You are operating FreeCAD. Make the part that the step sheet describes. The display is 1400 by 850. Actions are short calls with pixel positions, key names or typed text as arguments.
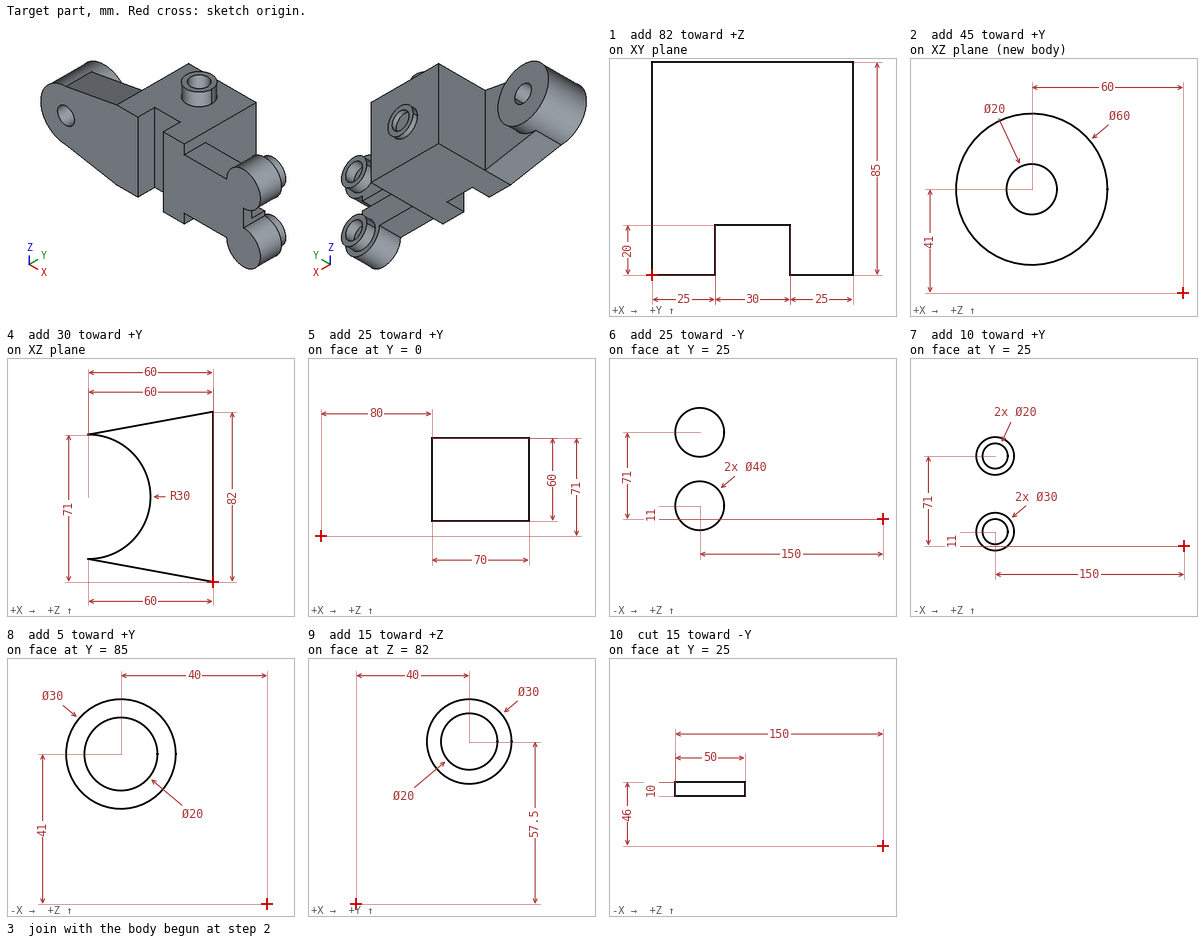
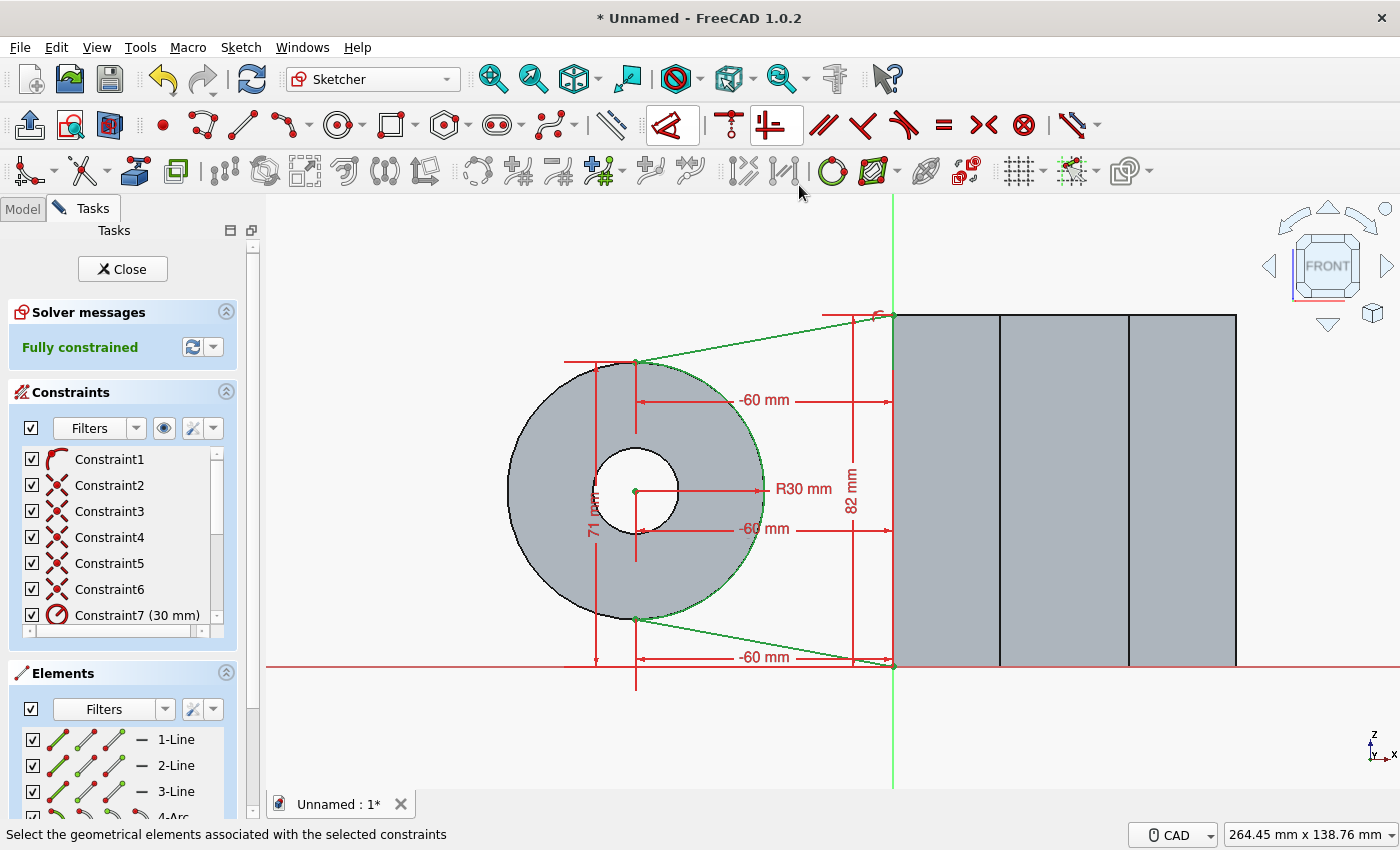
click(123, 269)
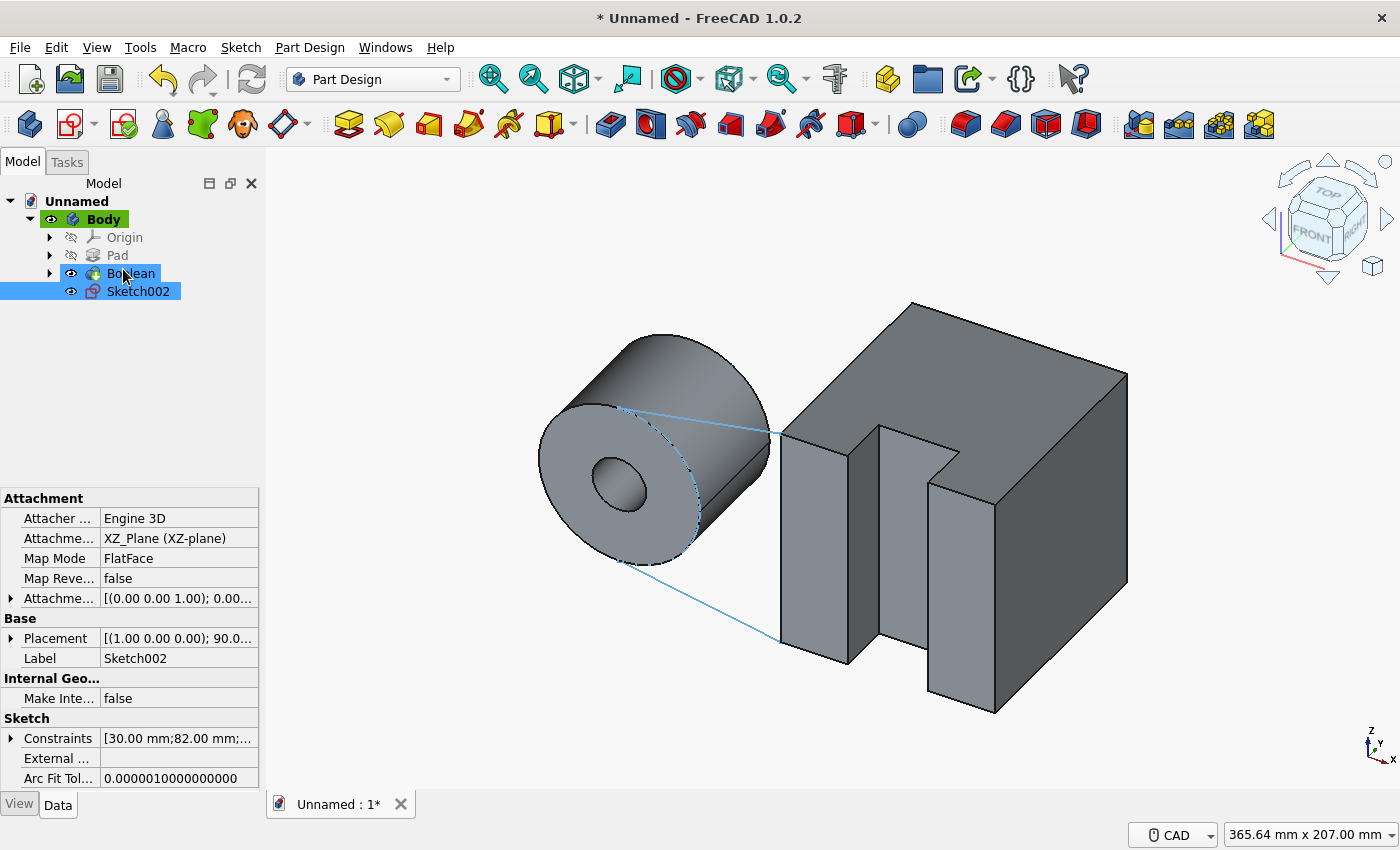
click(350, 124)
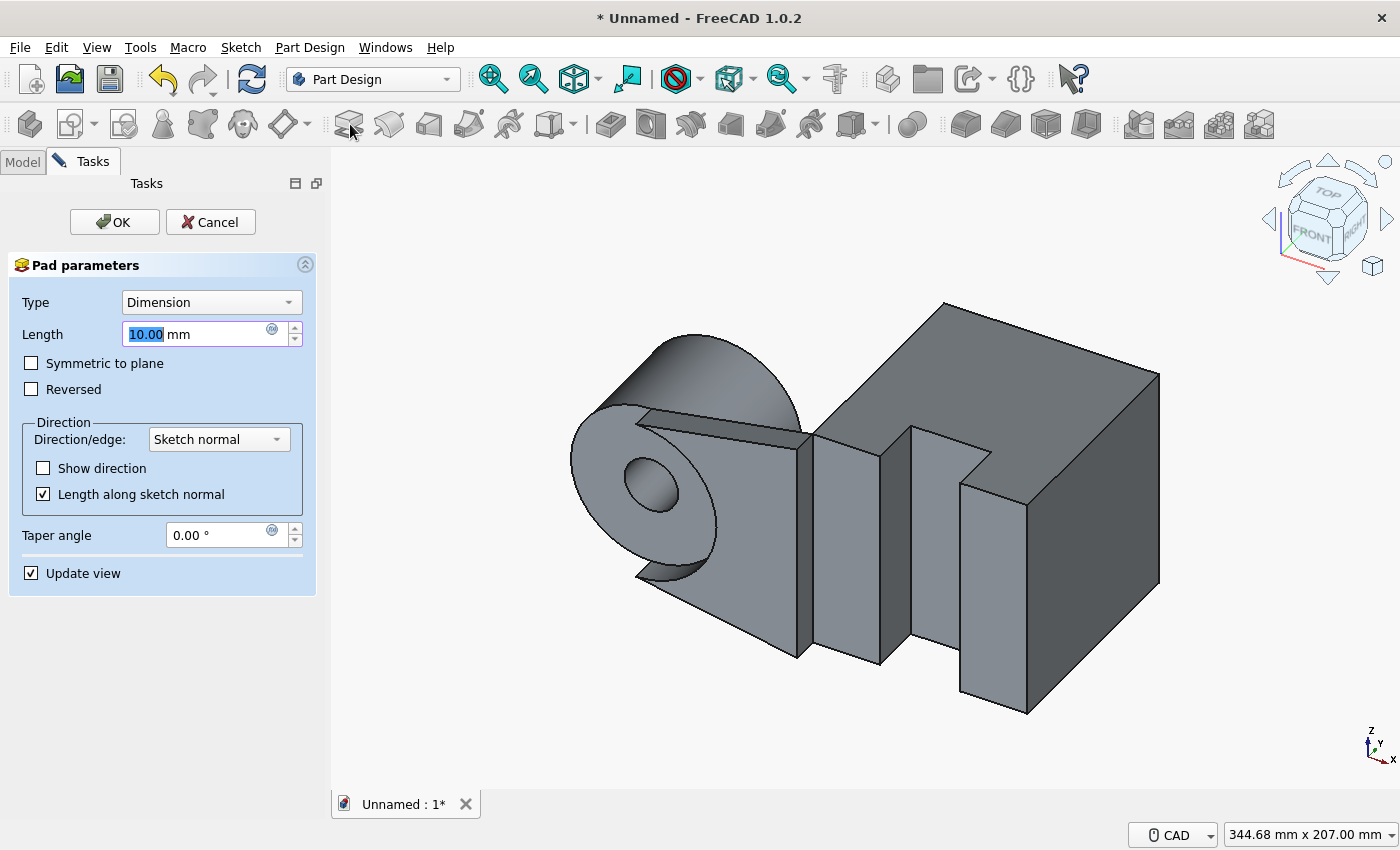
text(30)
key(Tab)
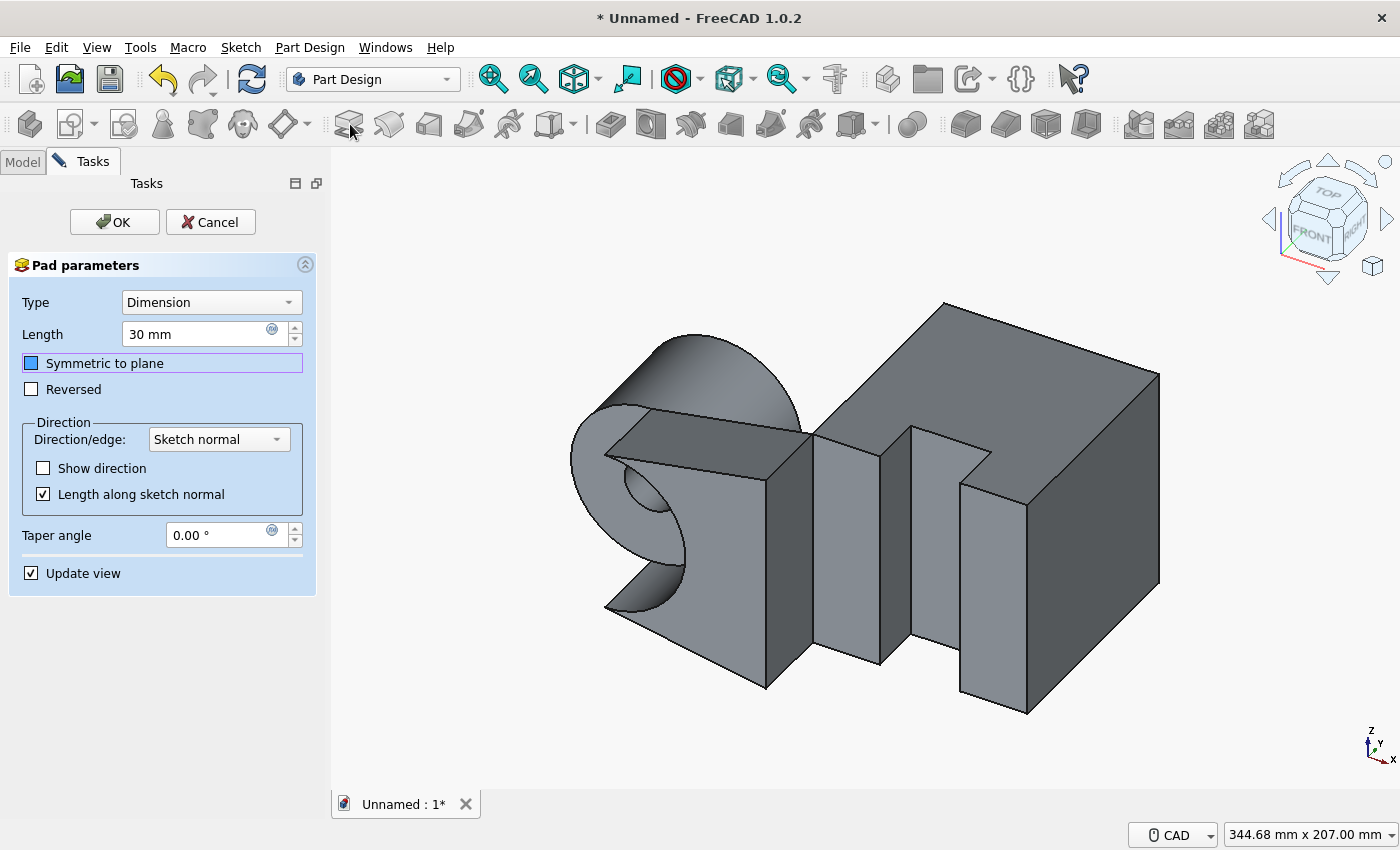
click(30, 389)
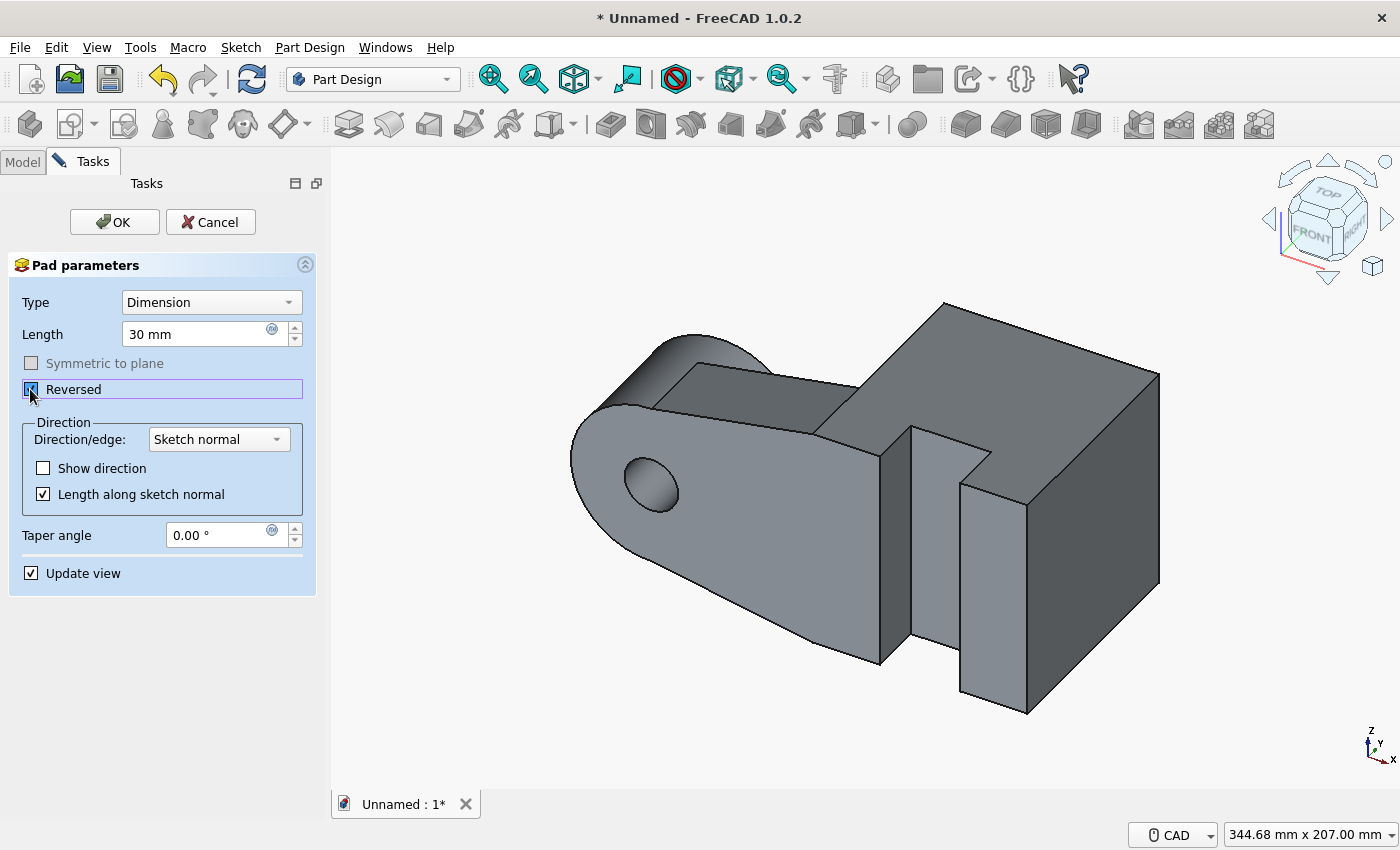
click(115, 222)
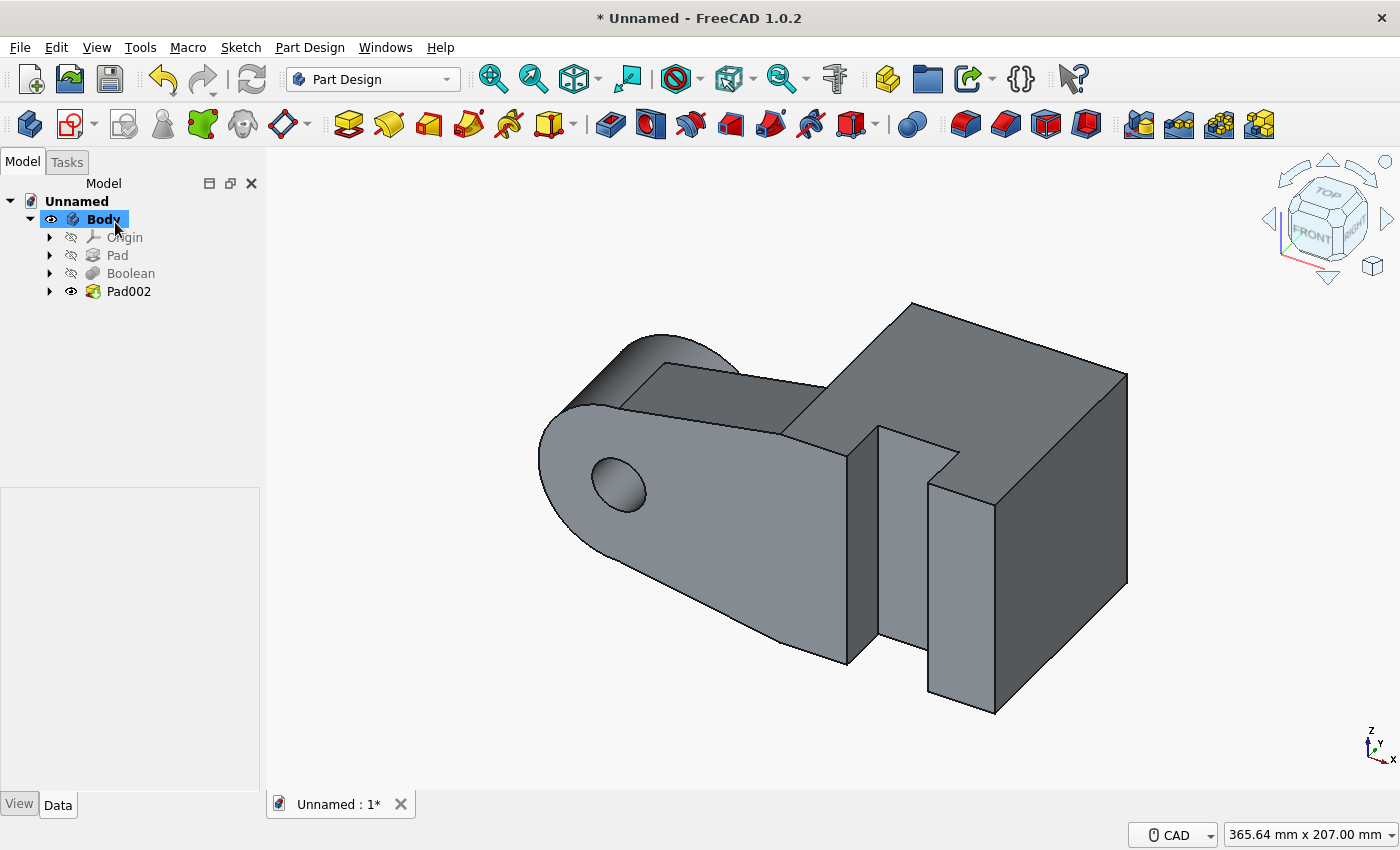
click(737, 523)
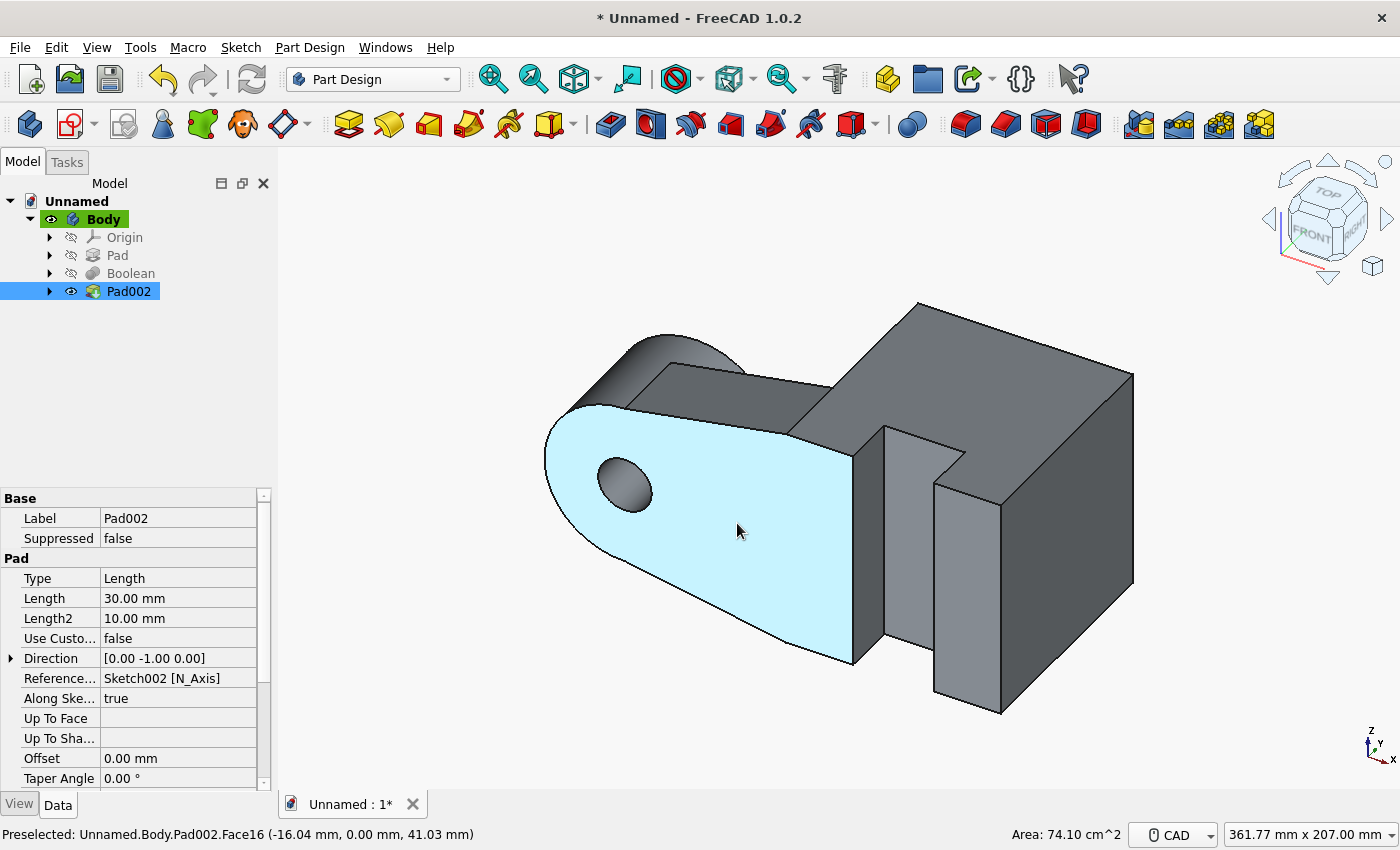
click(70, 124)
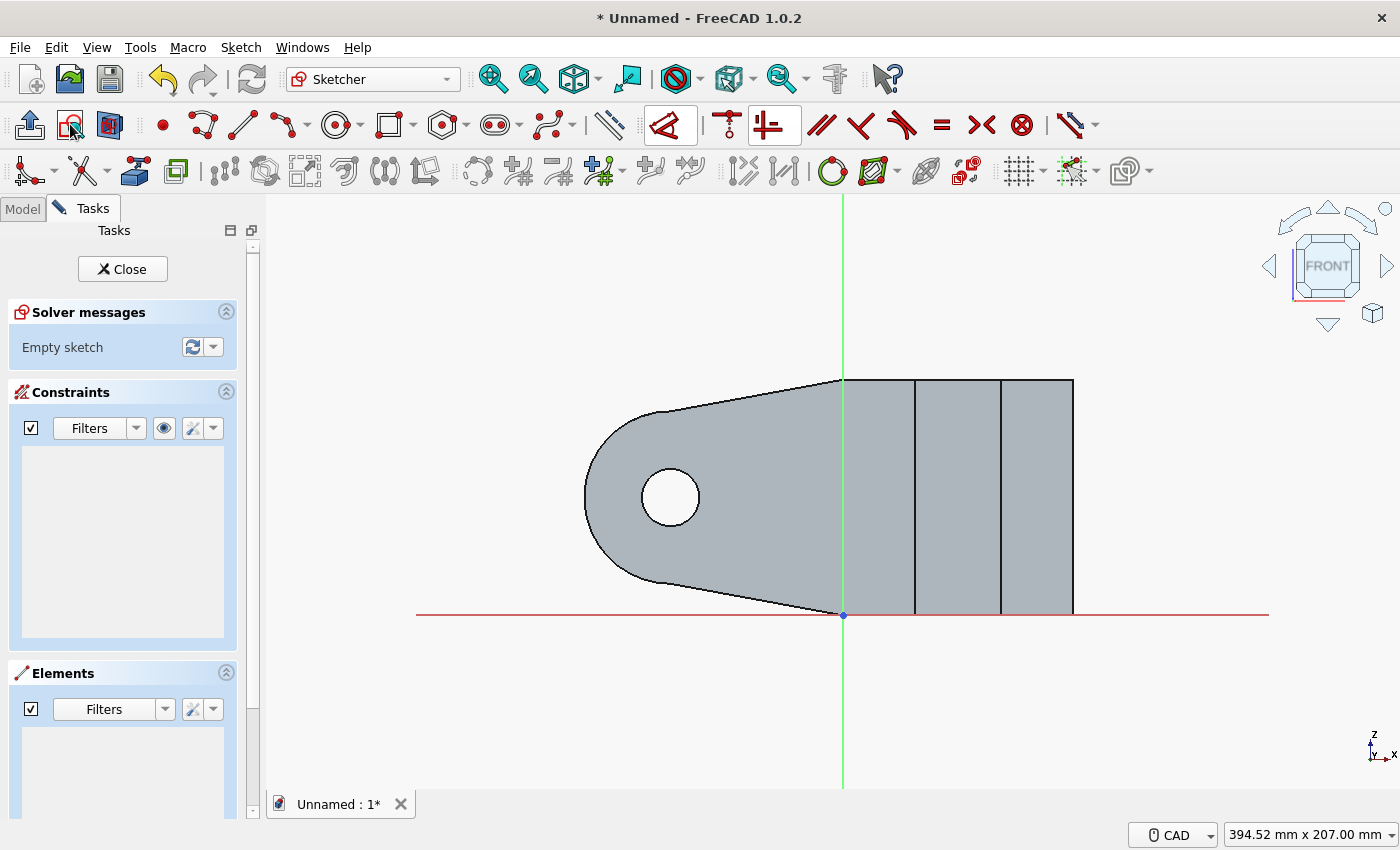
scroll(294, 393, down, 1)